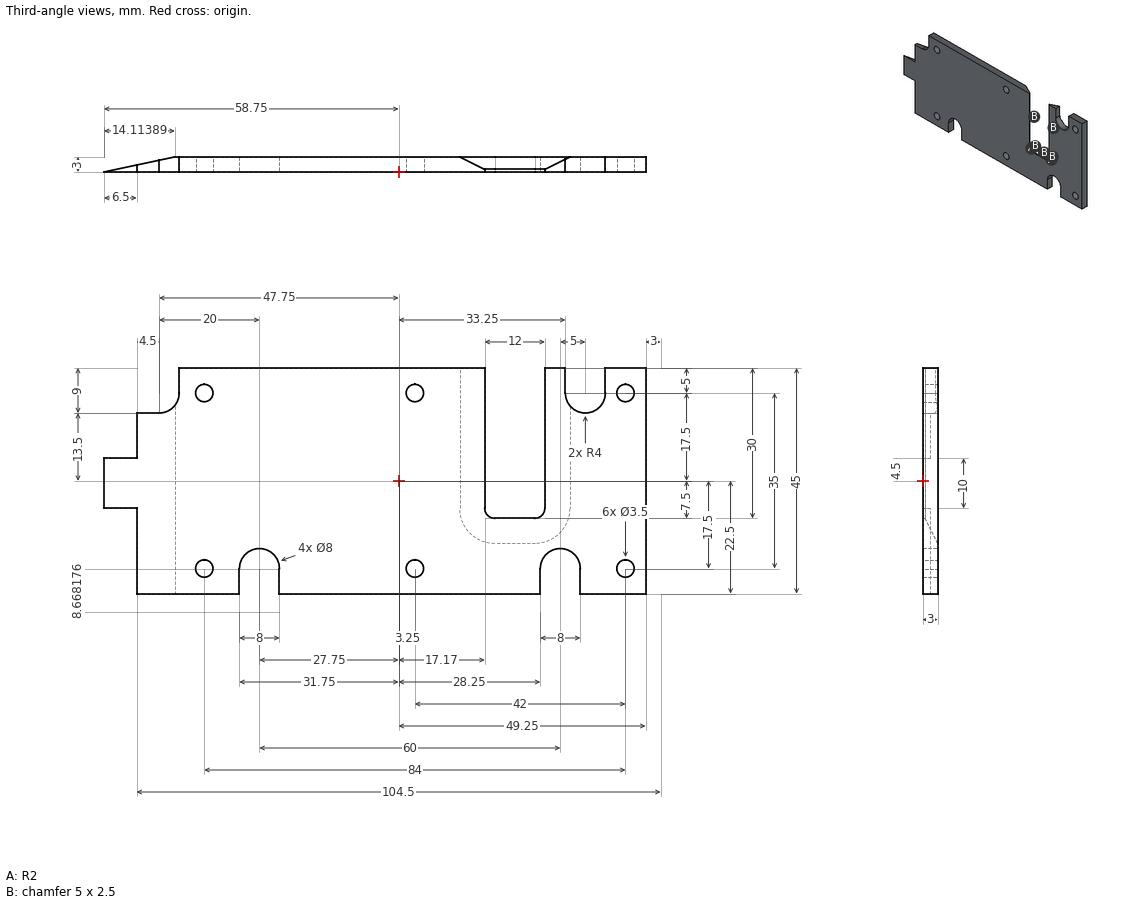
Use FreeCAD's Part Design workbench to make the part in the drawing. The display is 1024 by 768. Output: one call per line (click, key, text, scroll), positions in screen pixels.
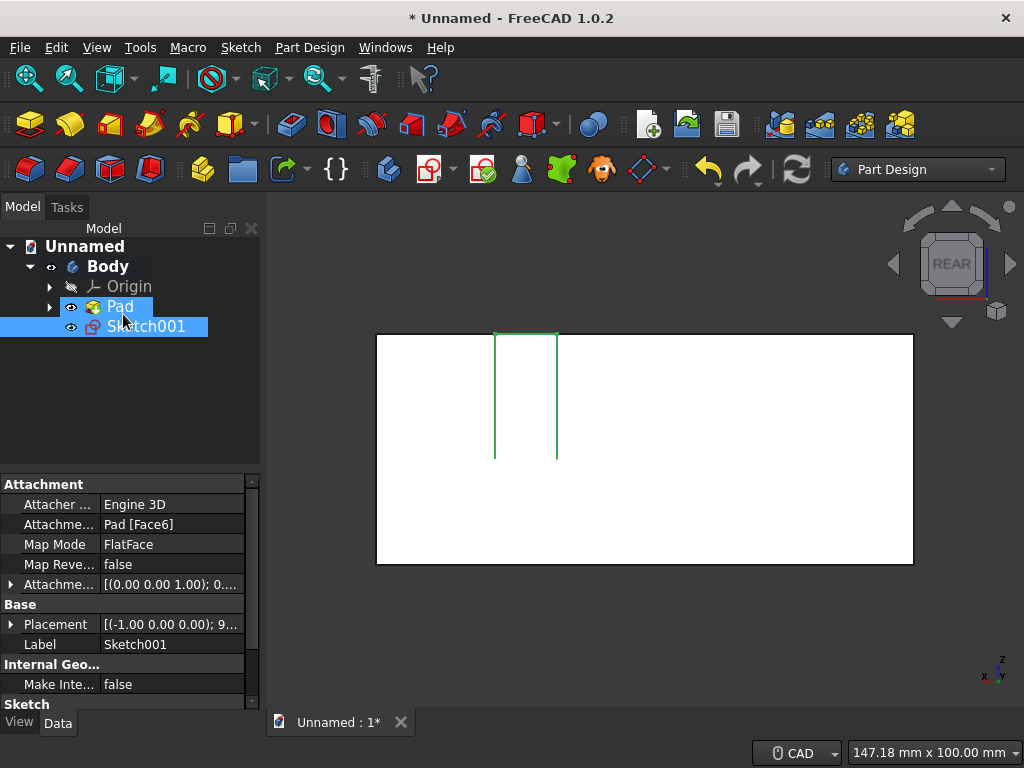
click(292, 124)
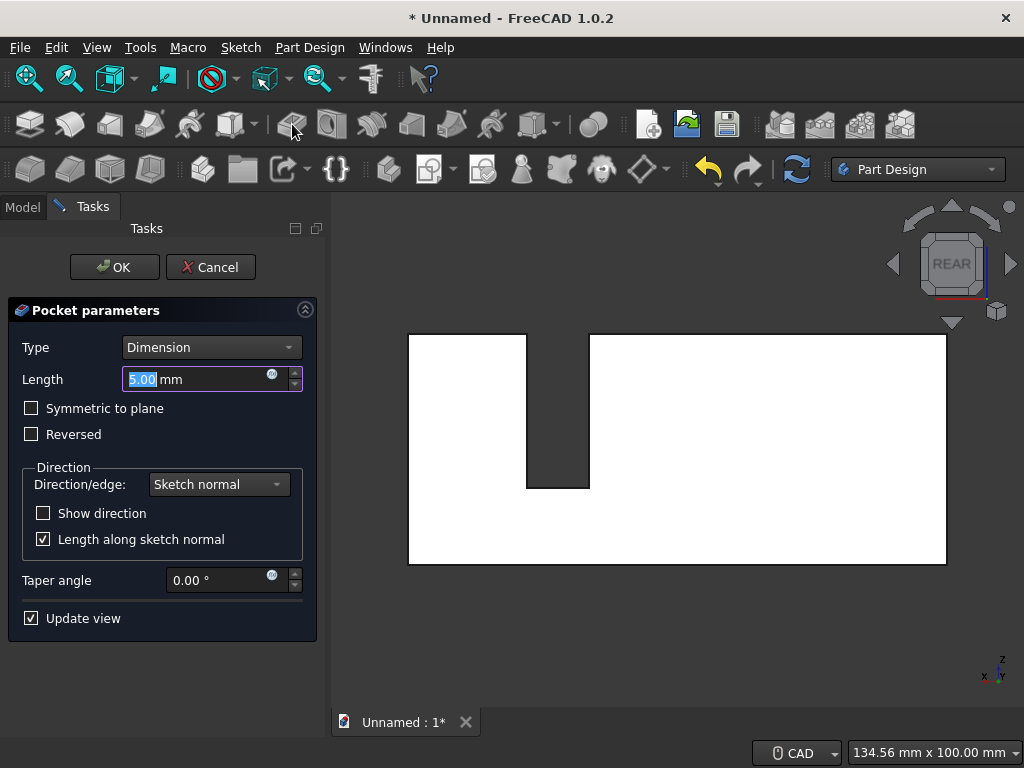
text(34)
key(Tab)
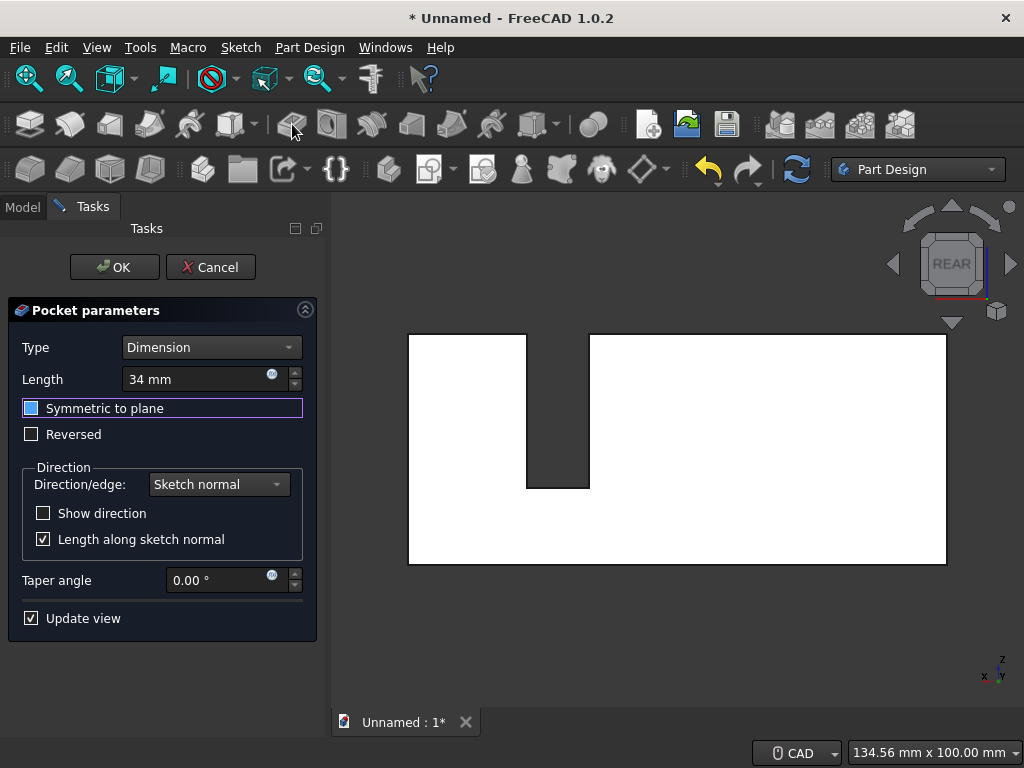
click(115, 267)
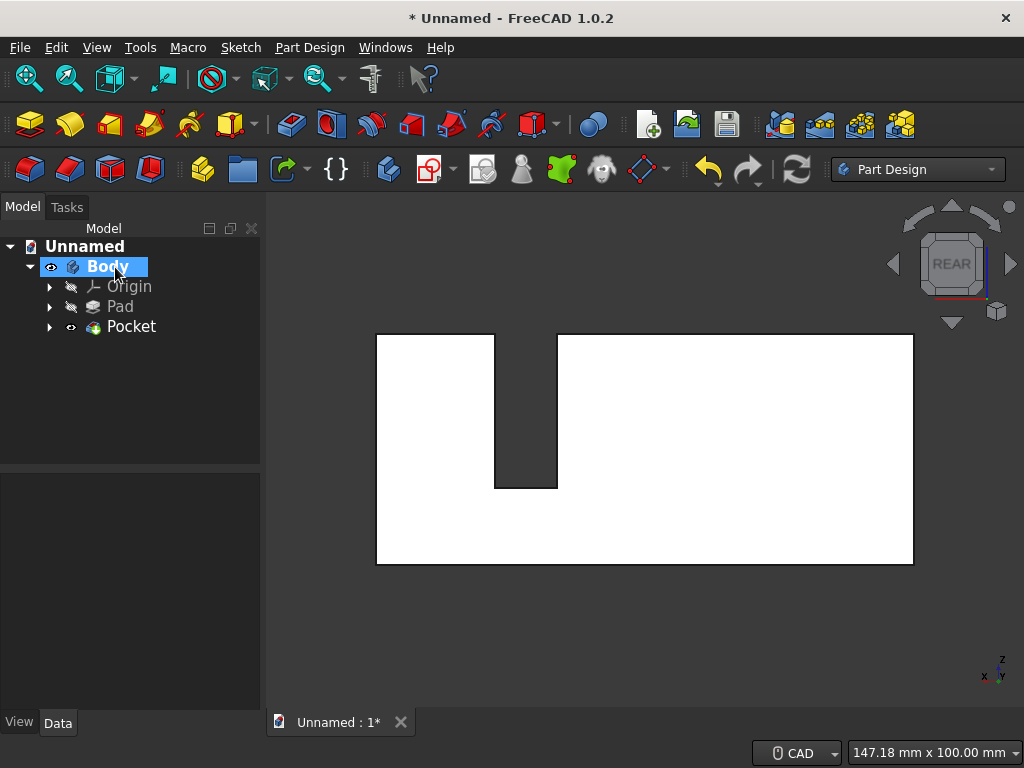
click(722, 448)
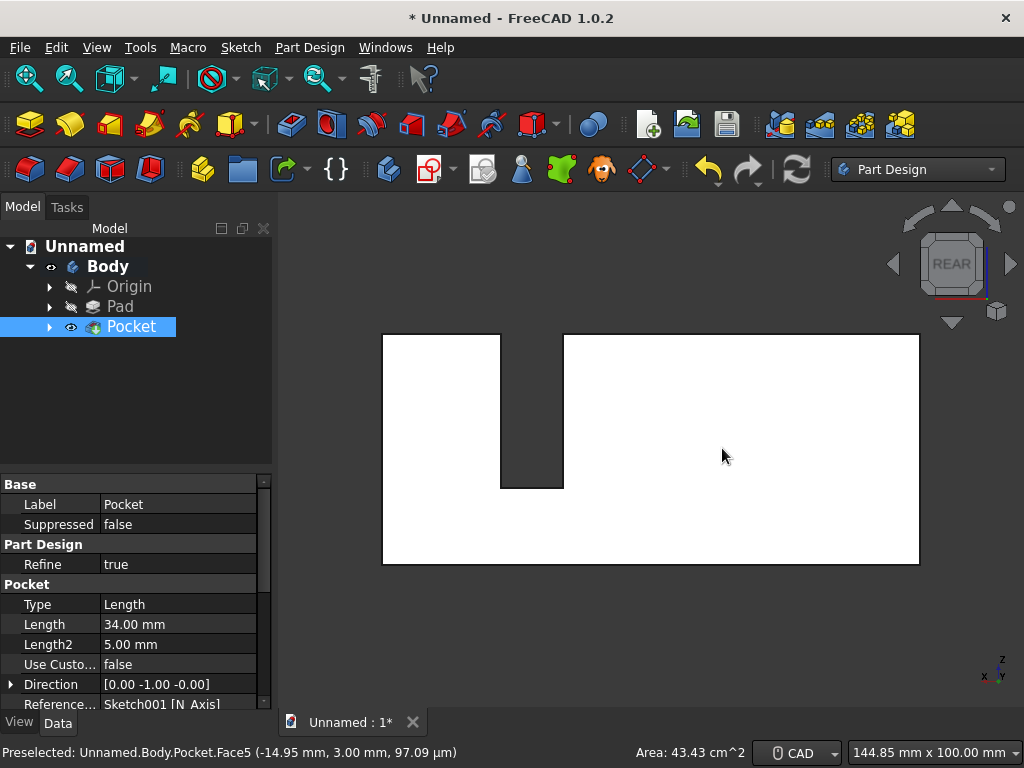
click(430, 170)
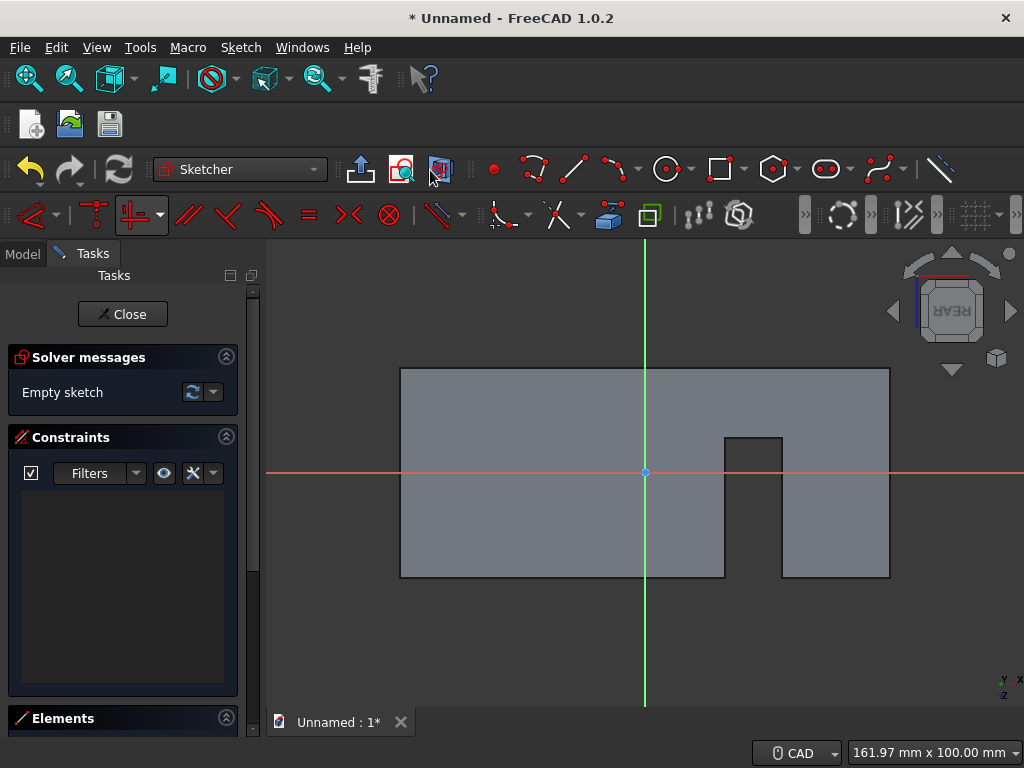
scroll(294, 473, down, 1)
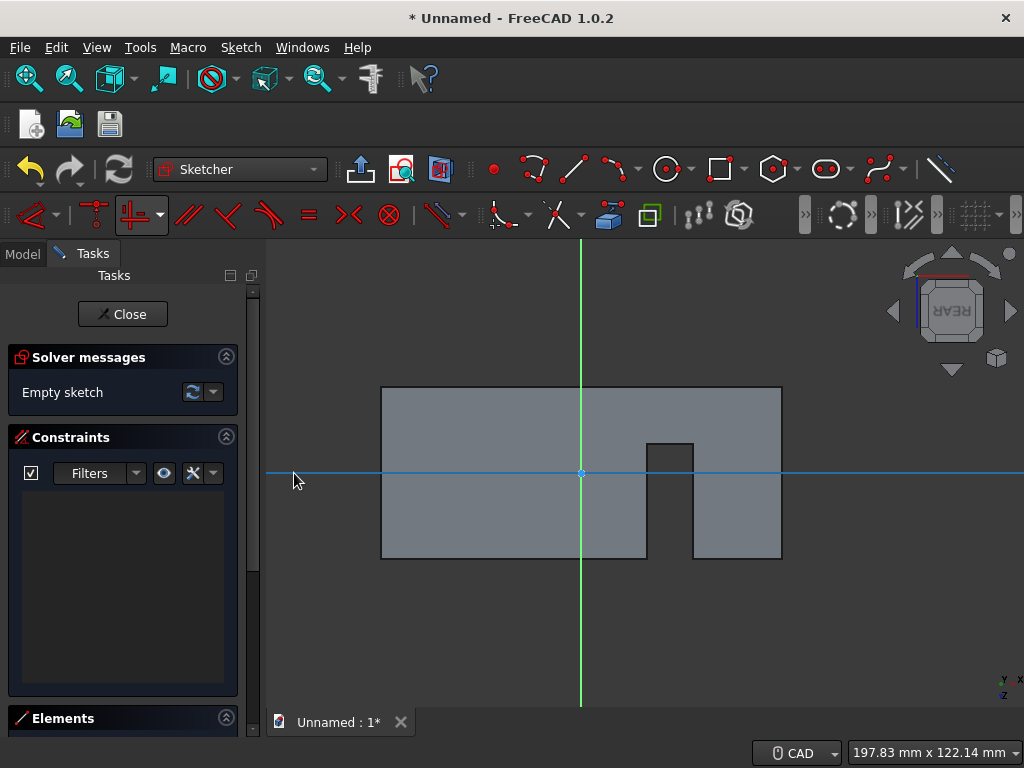
scroll(809, 473, up, 3)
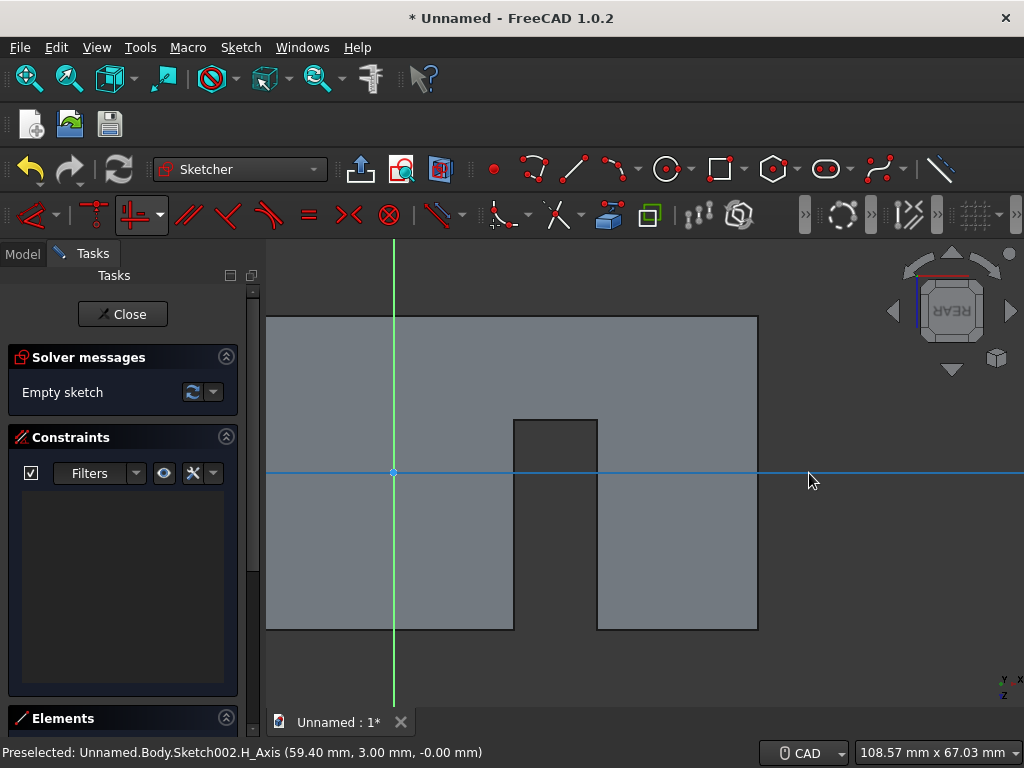
click(720, 170)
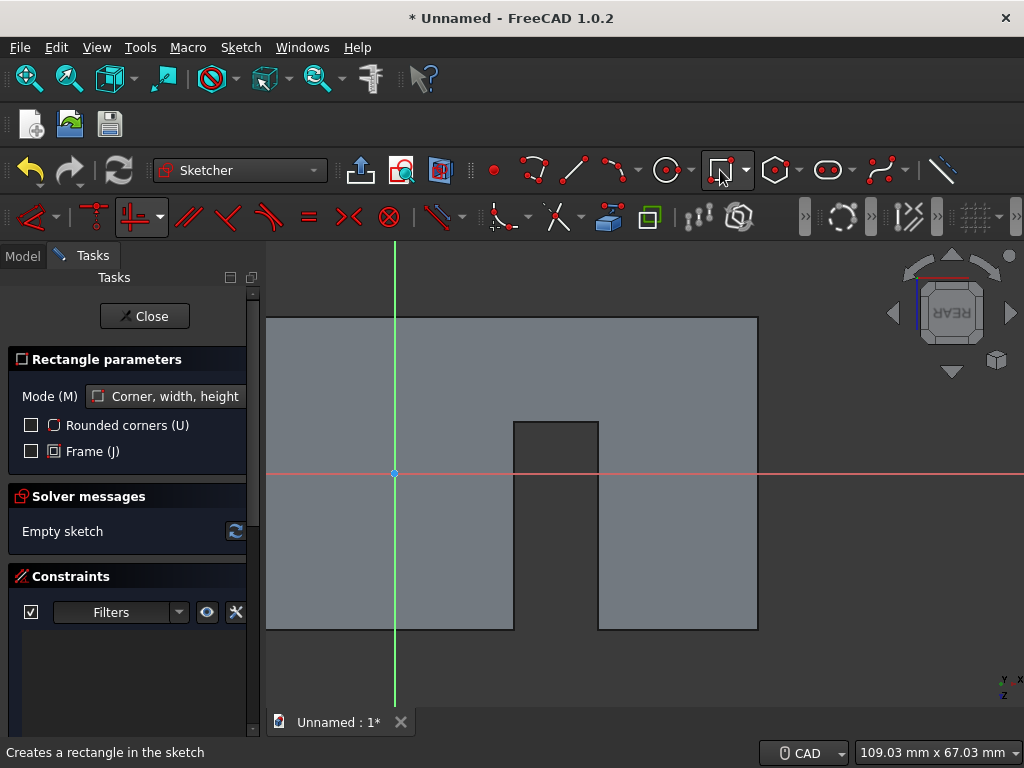
click(737, 317)
move(758, 630)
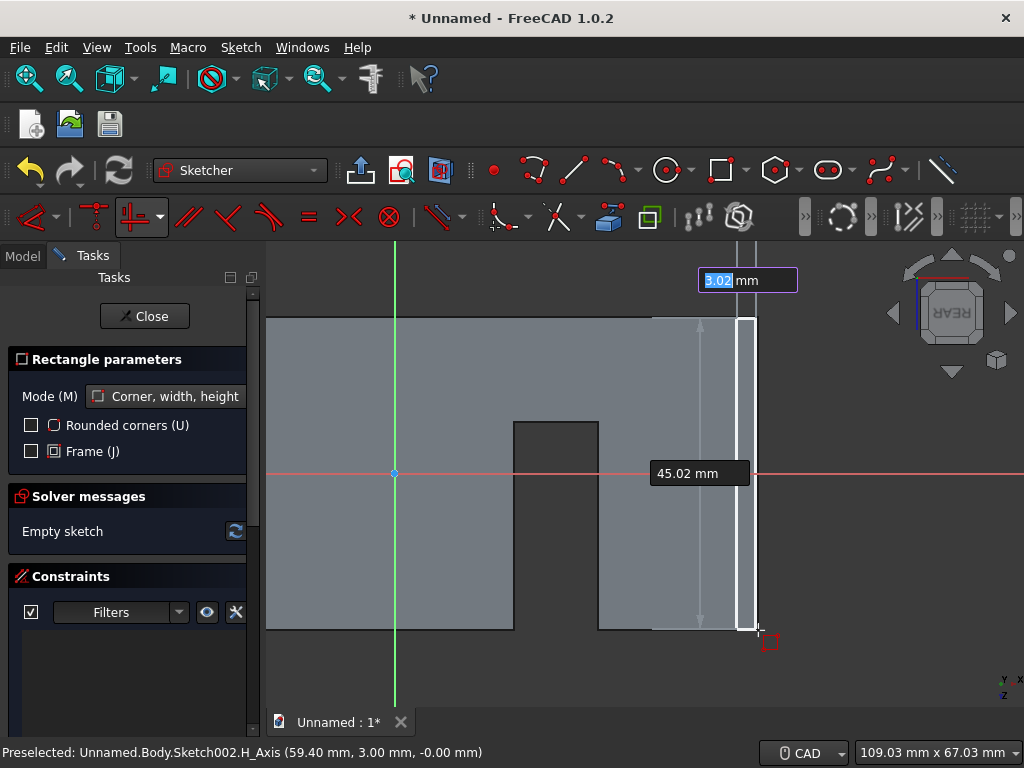
text(3)
key(Tab)
text(45)
key(Return)
key(Escape)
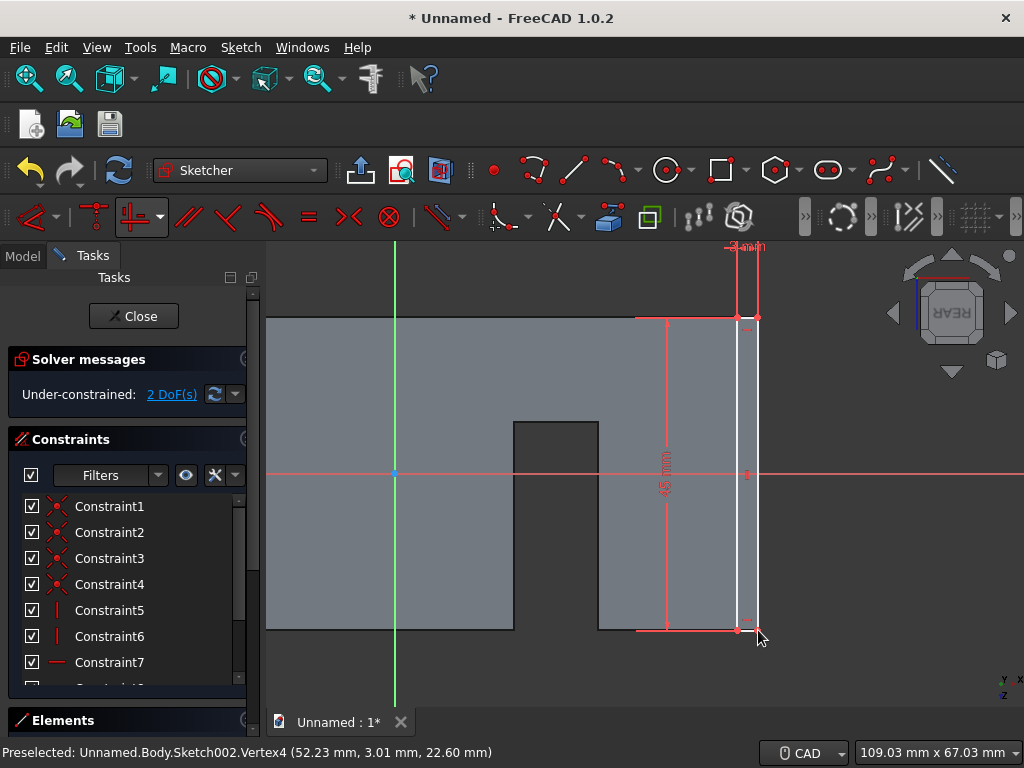
key(d)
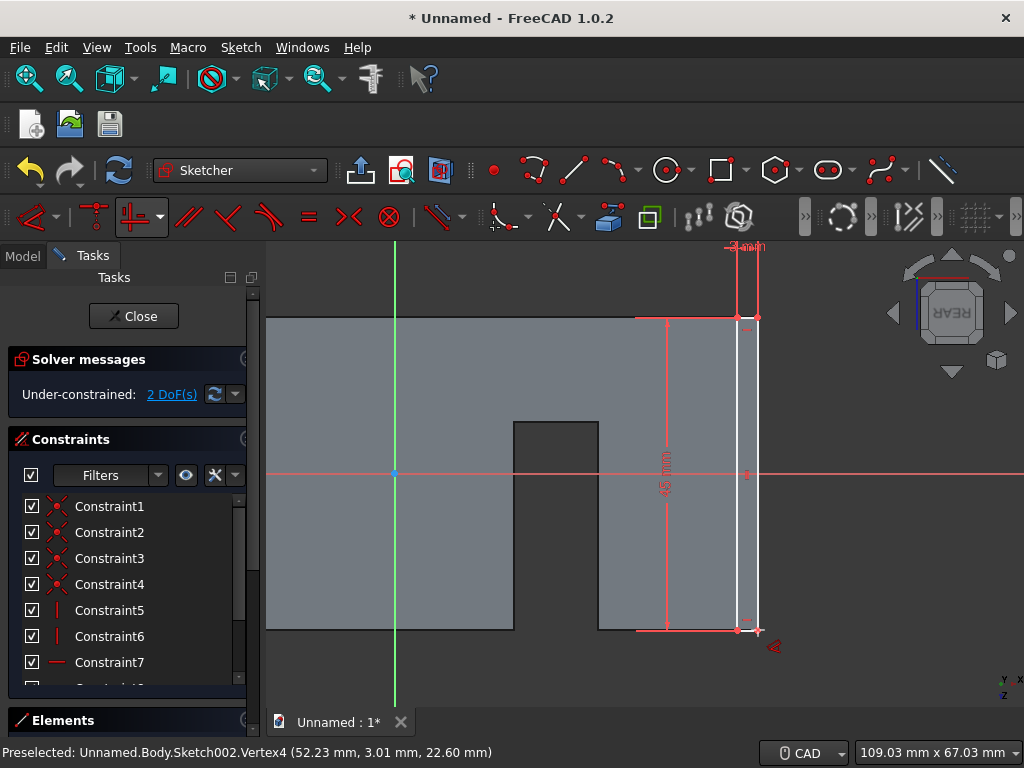
click(737, 318)
click(361, 396)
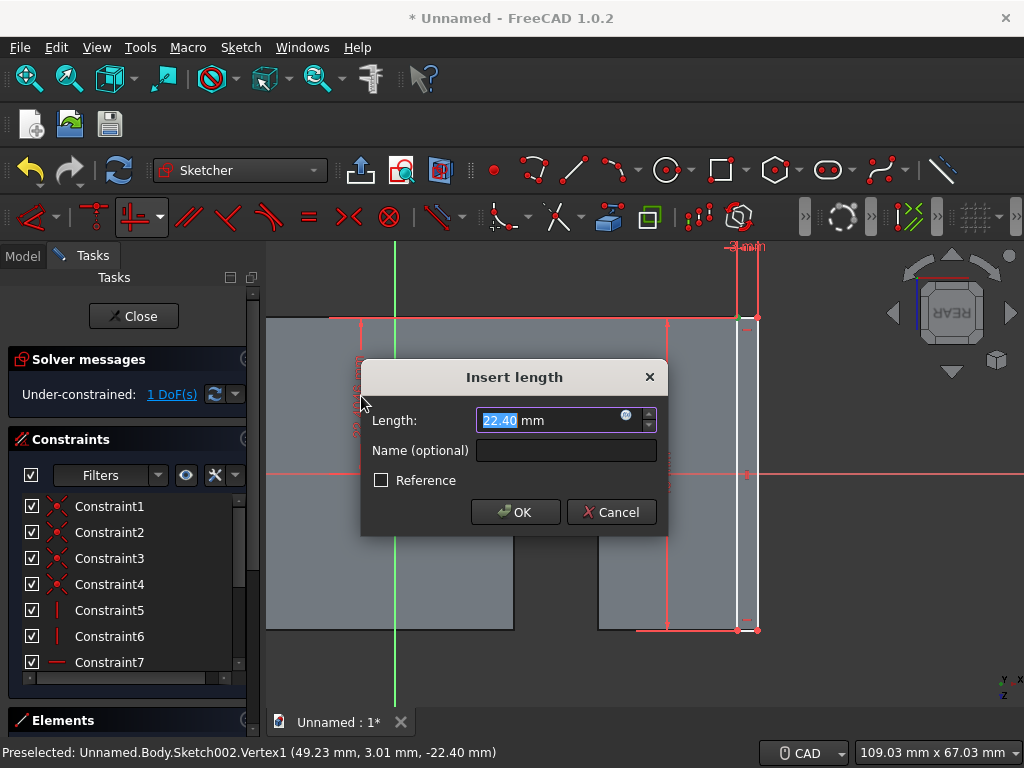
text(22.5)
key(Return)